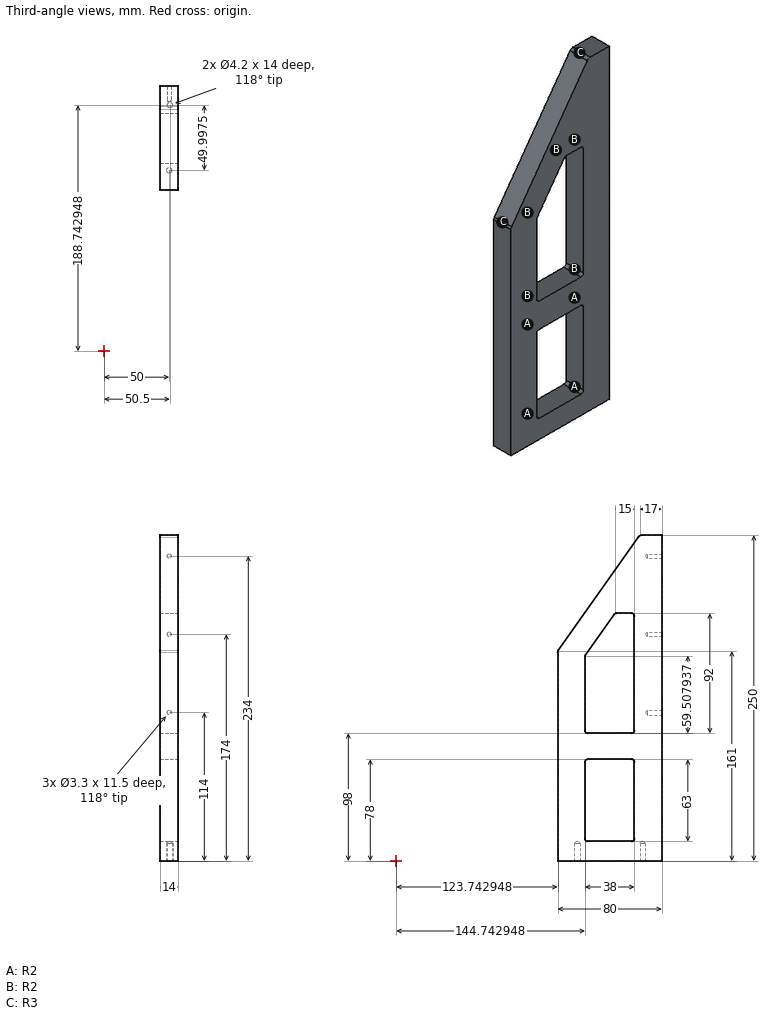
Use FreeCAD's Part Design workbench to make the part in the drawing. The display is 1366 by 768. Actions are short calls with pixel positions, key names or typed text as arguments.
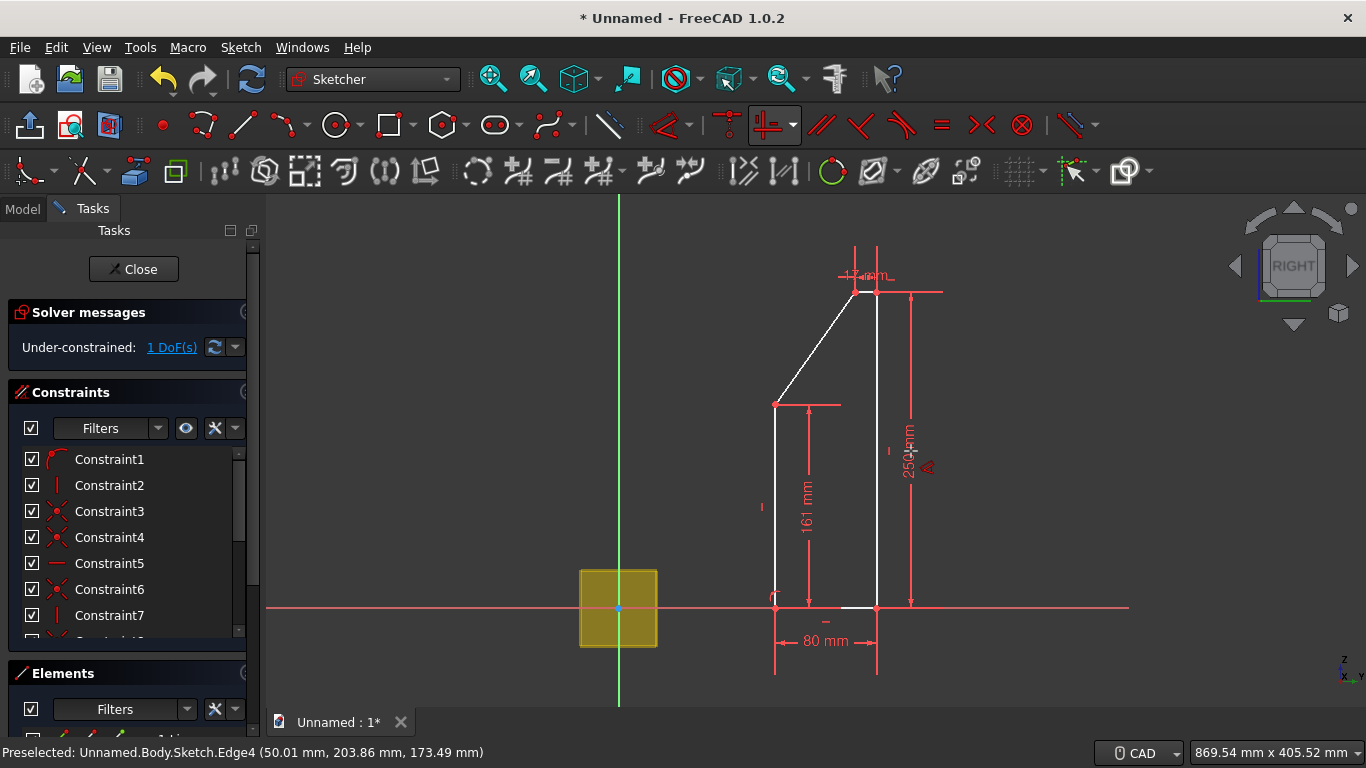
click(775, 608)
click(697, 642)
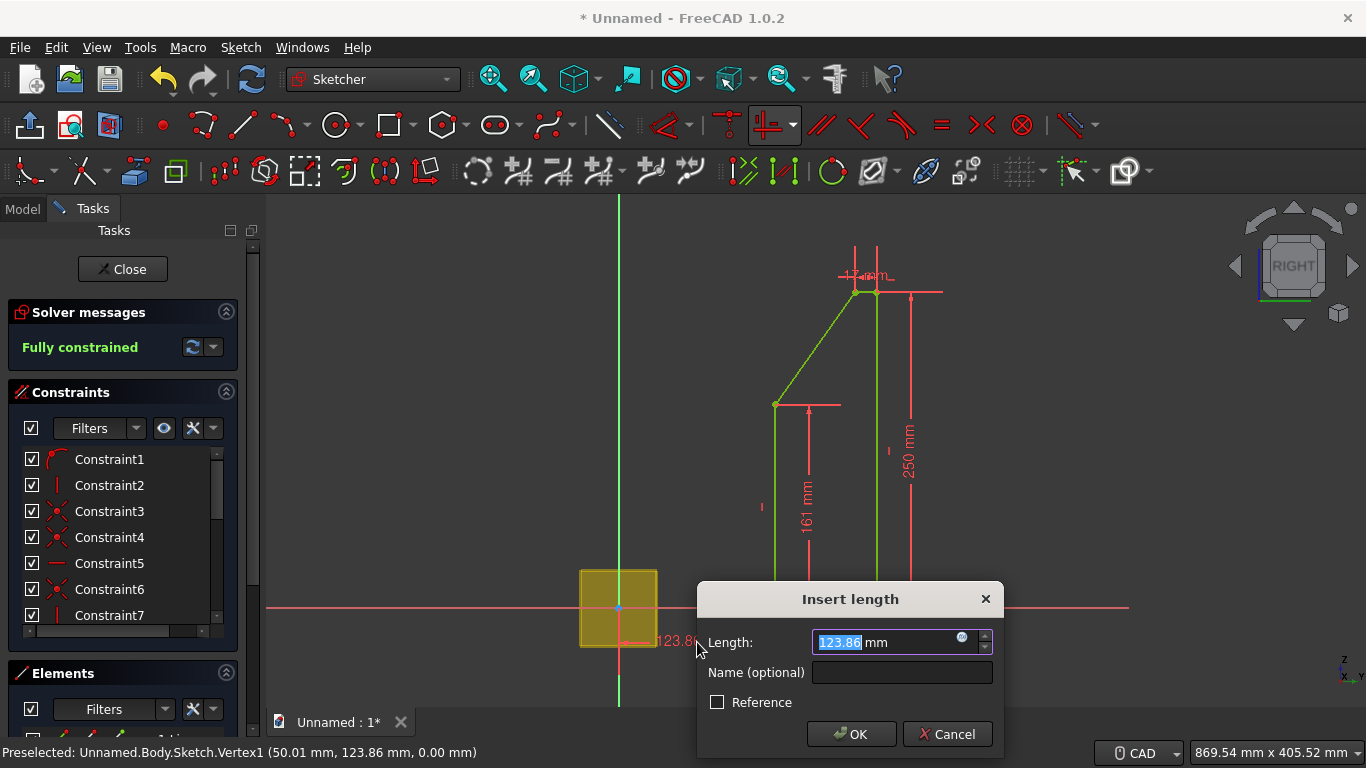
text(123.742948)
key(Return)
key(Escape)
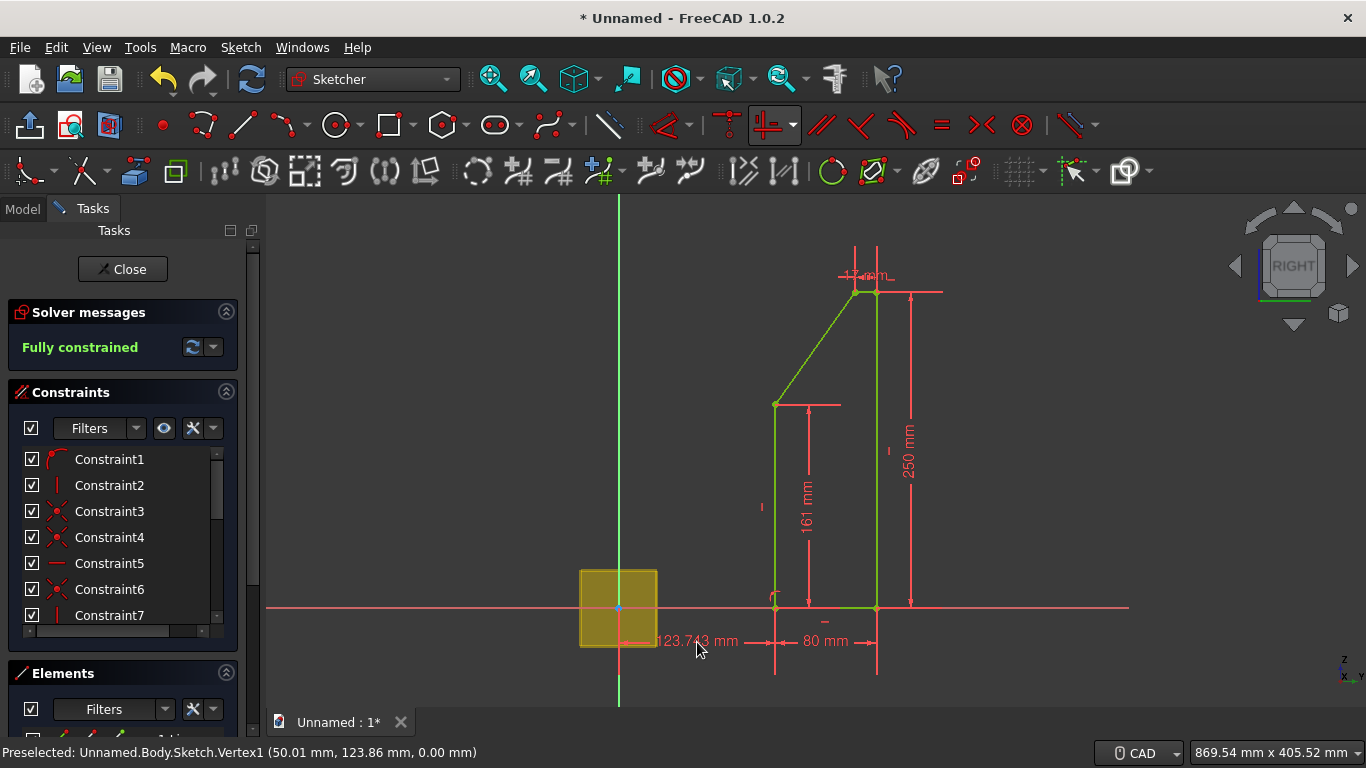
click(123, 269)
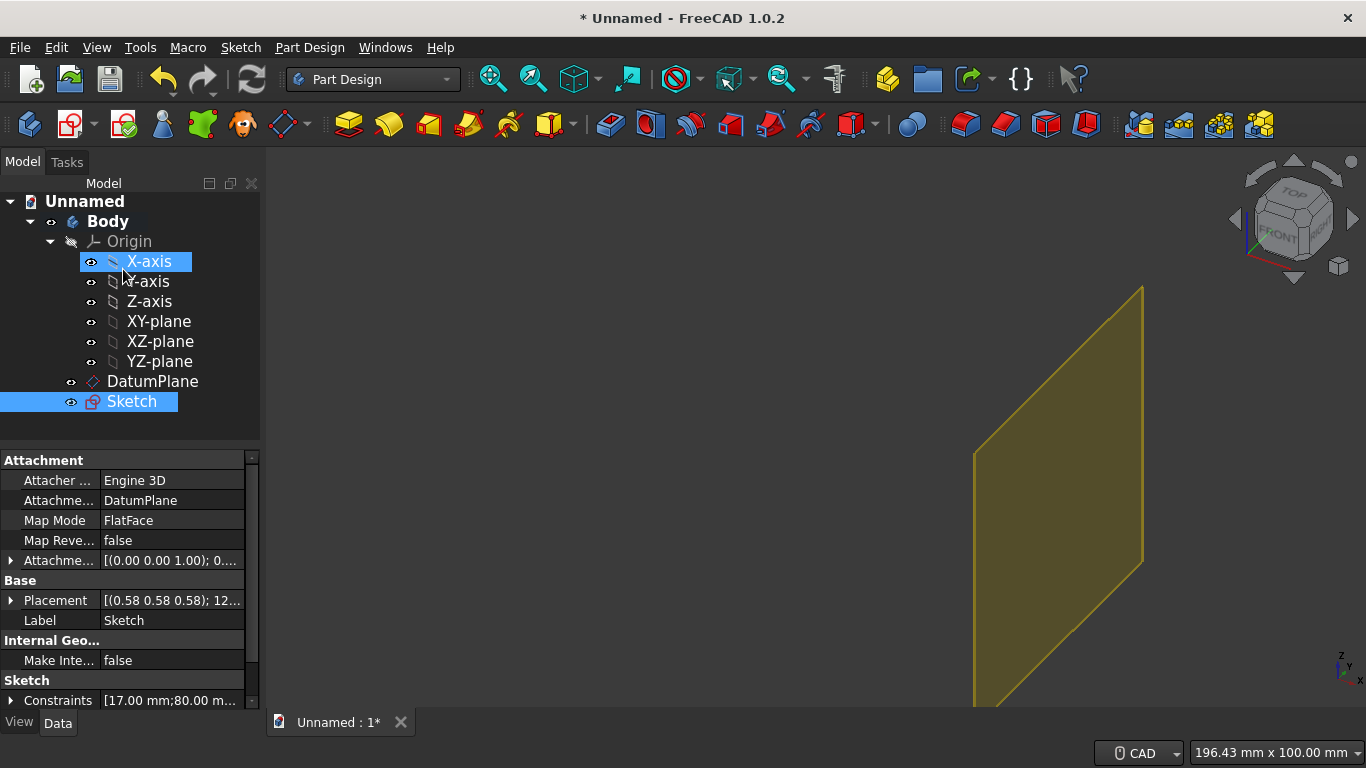
click(350, 124)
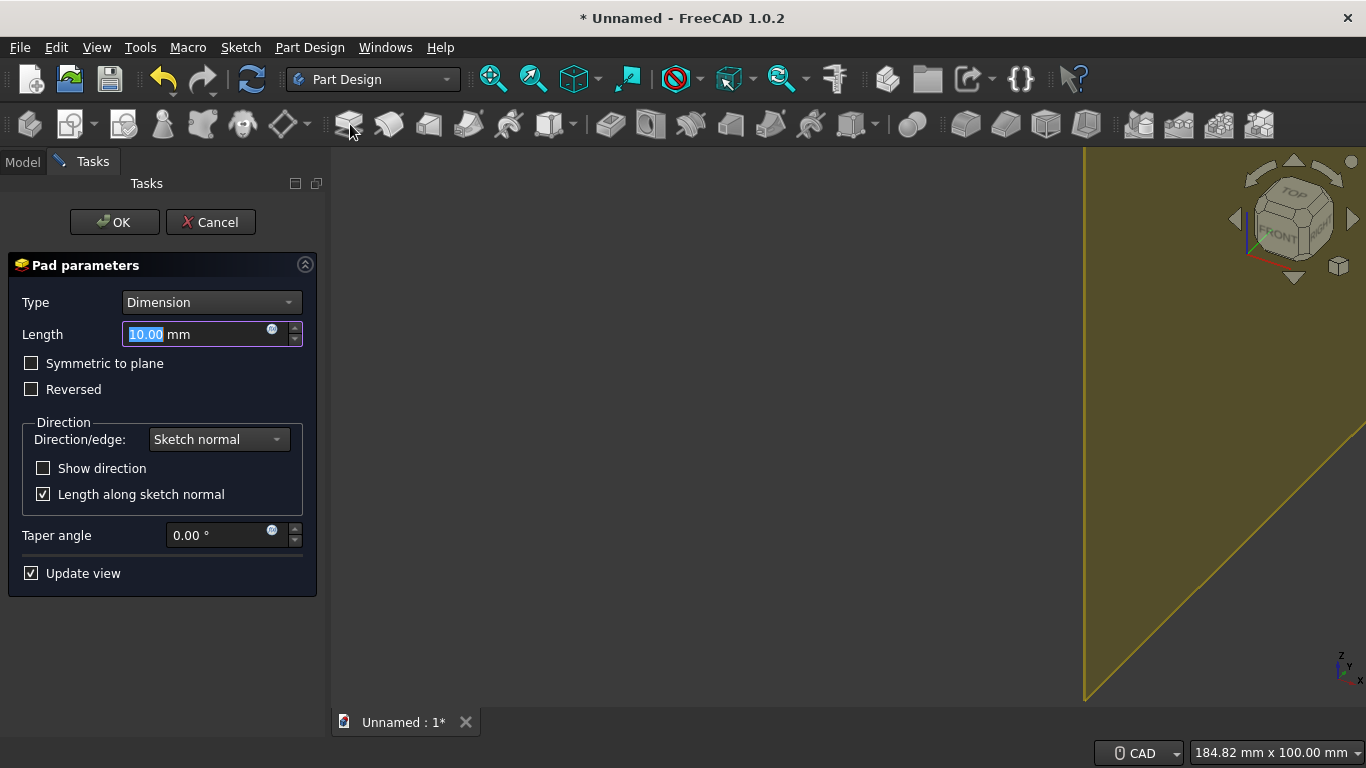
text(14)
key(Tab)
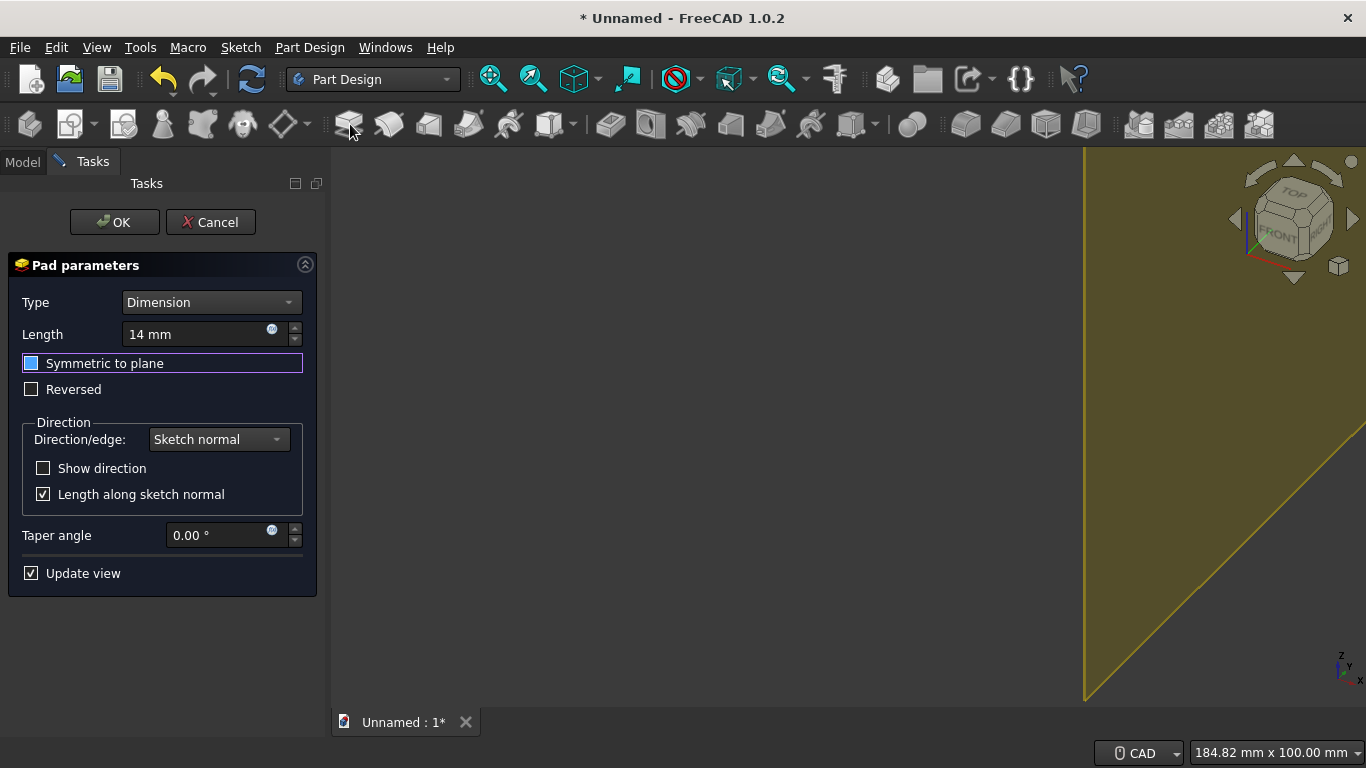
click(30, 363)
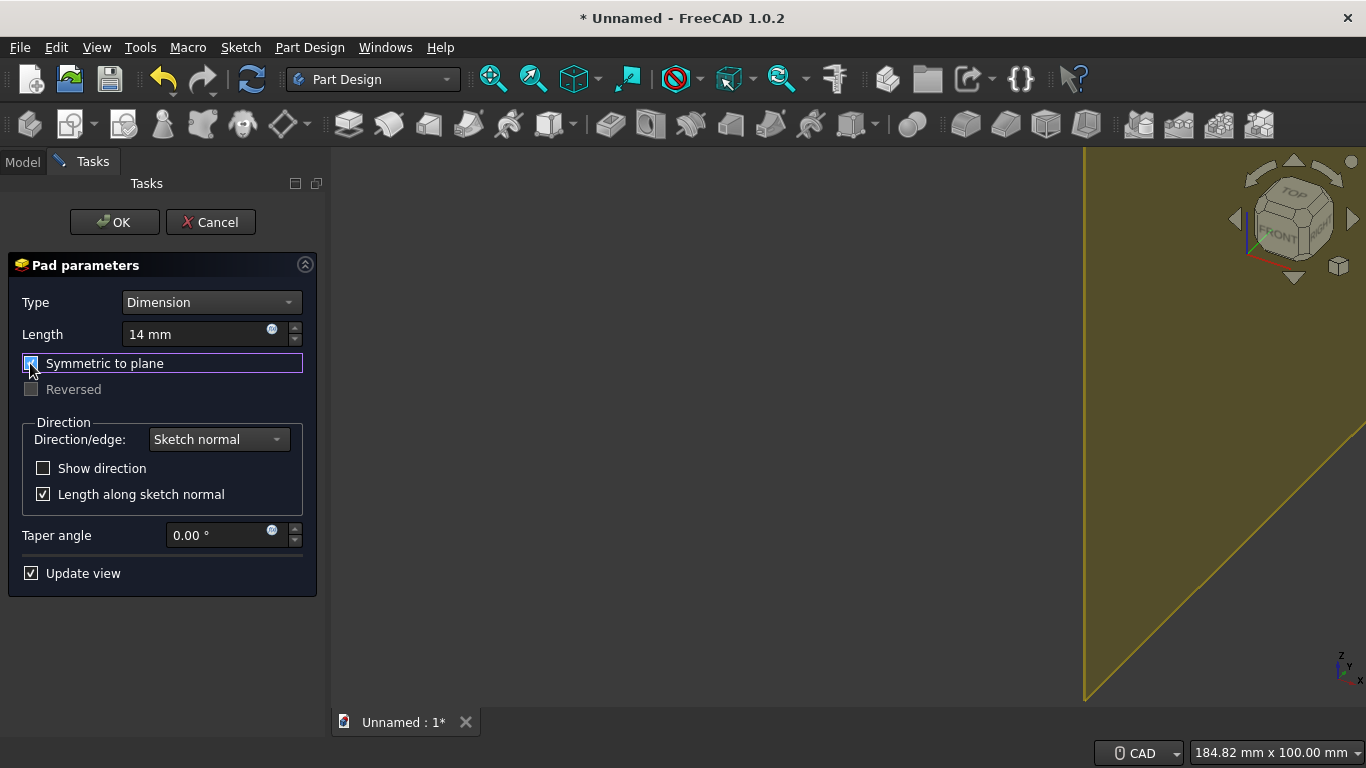
click(115, 222)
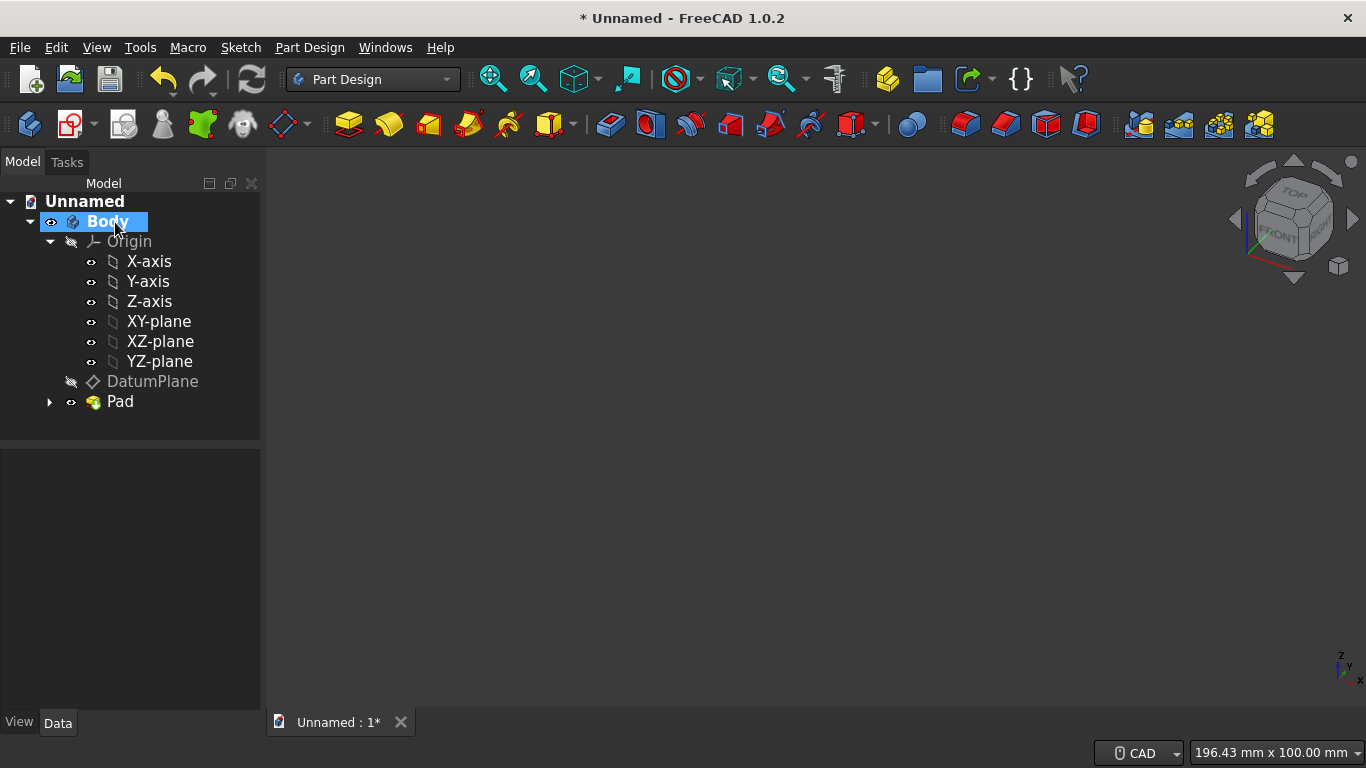
click(494, 80)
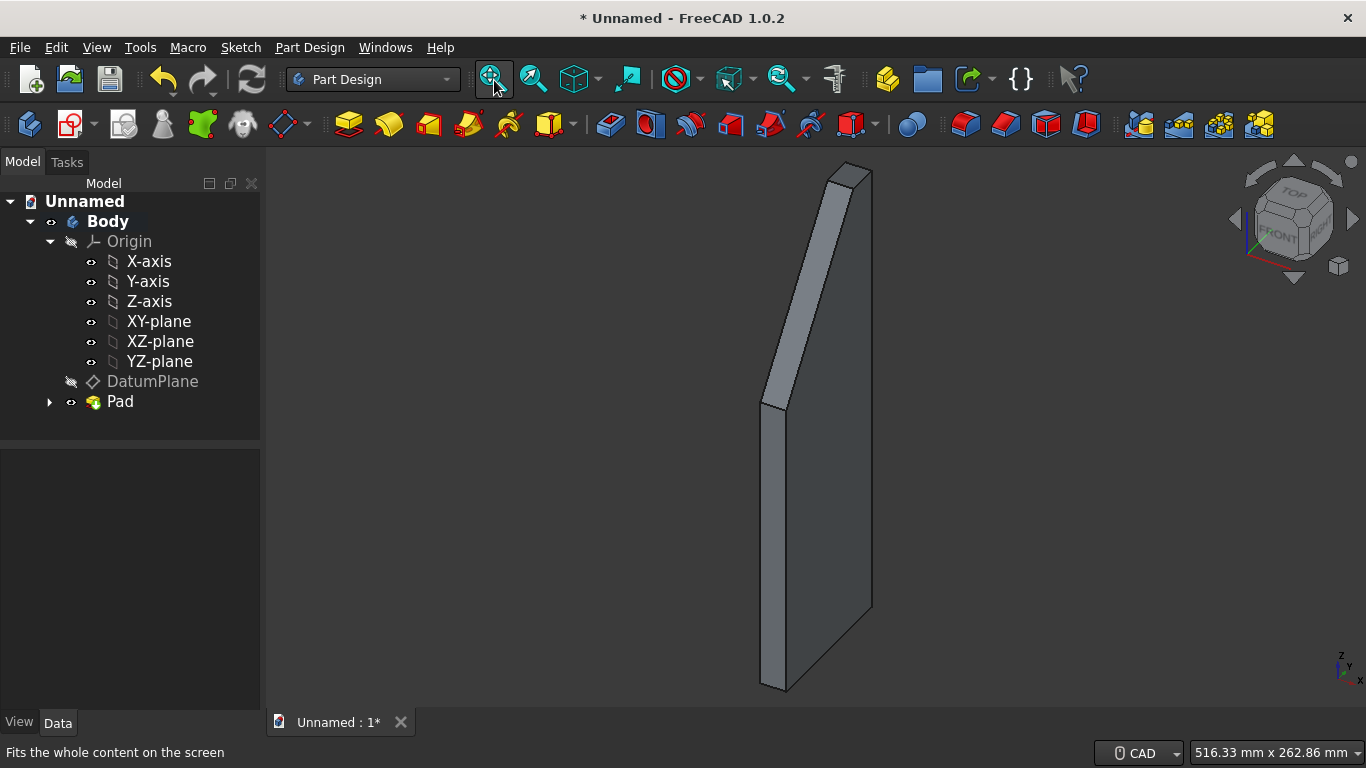
click(829, 555)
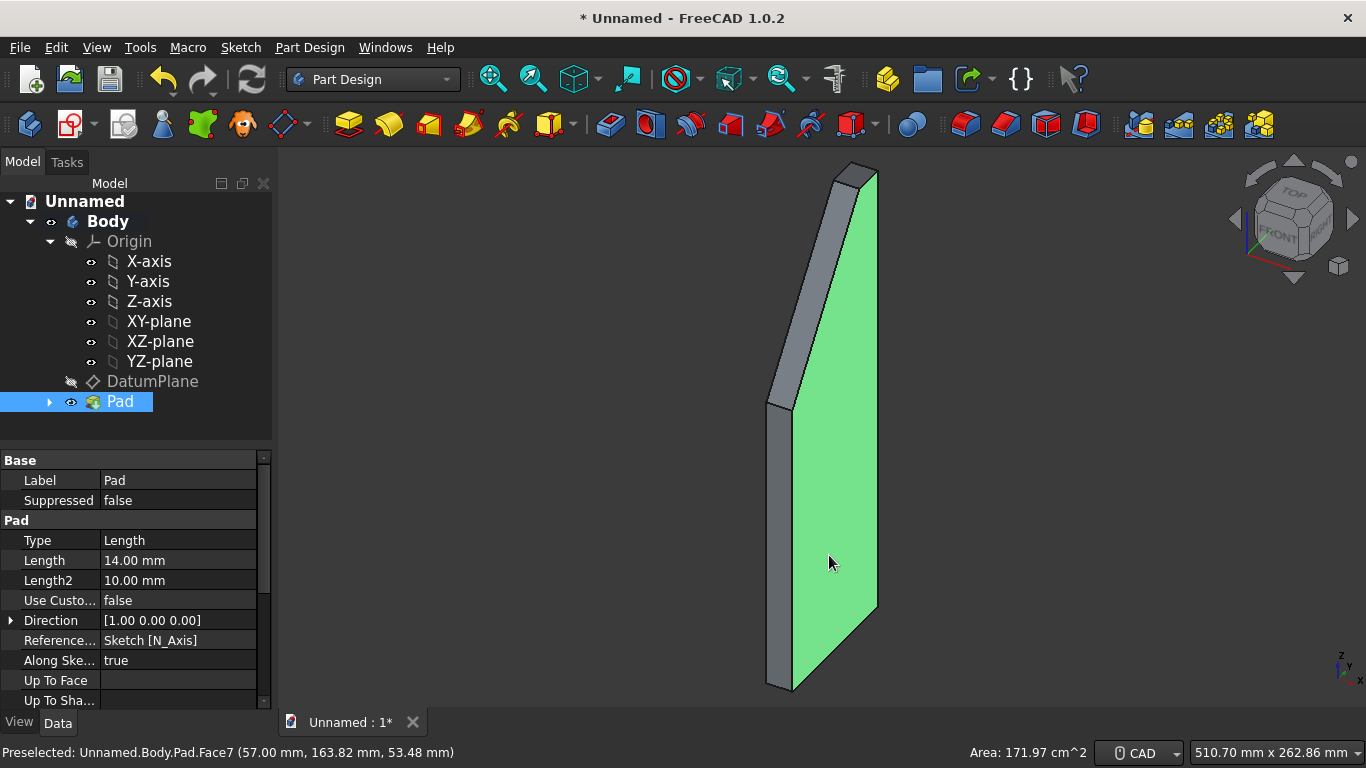
click(70, 124)